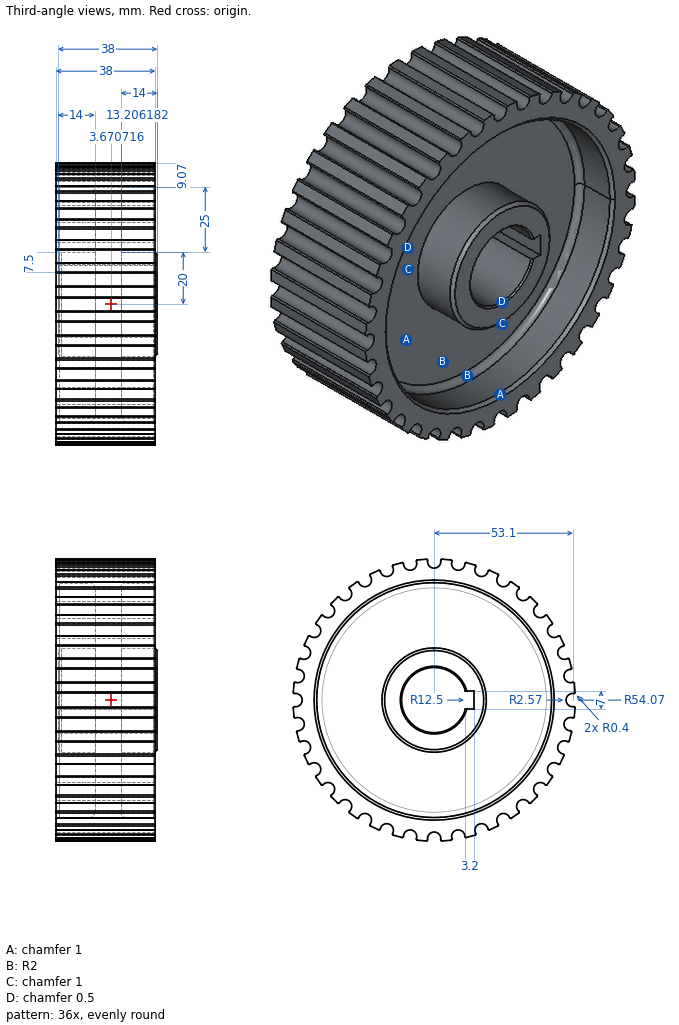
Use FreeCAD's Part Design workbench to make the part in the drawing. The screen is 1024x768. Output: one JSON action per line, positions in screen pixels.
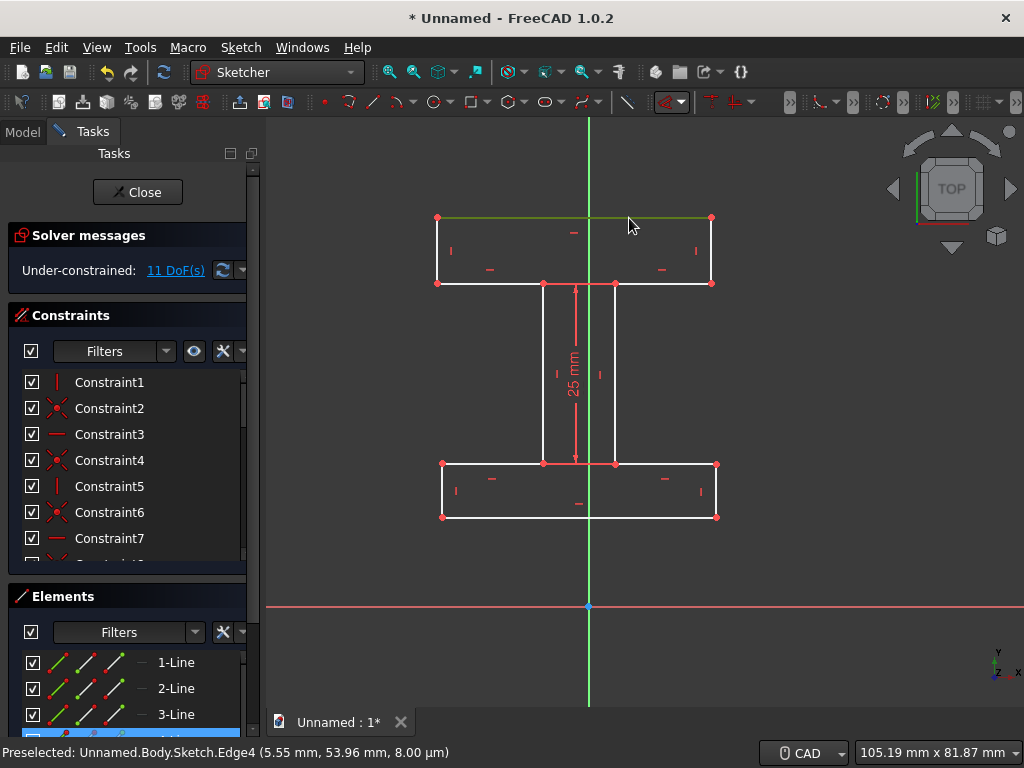
{"action": "left_click", "coordinate": [684, 102]}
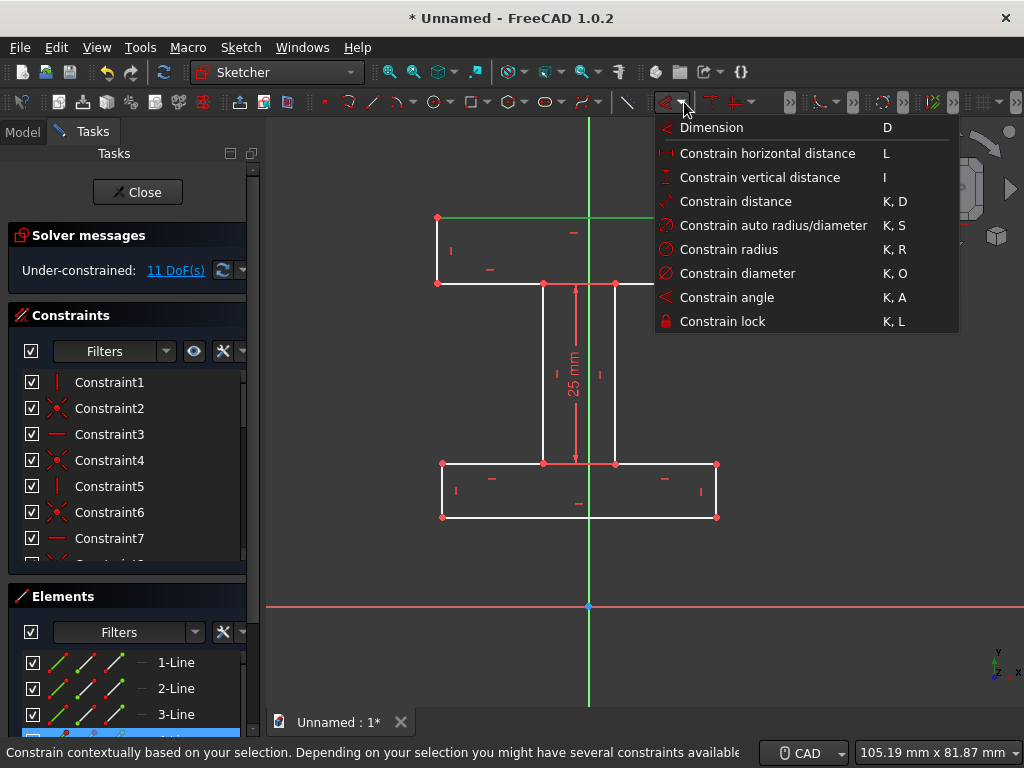
{"action": "left_click", "coordinate": [807, 153]}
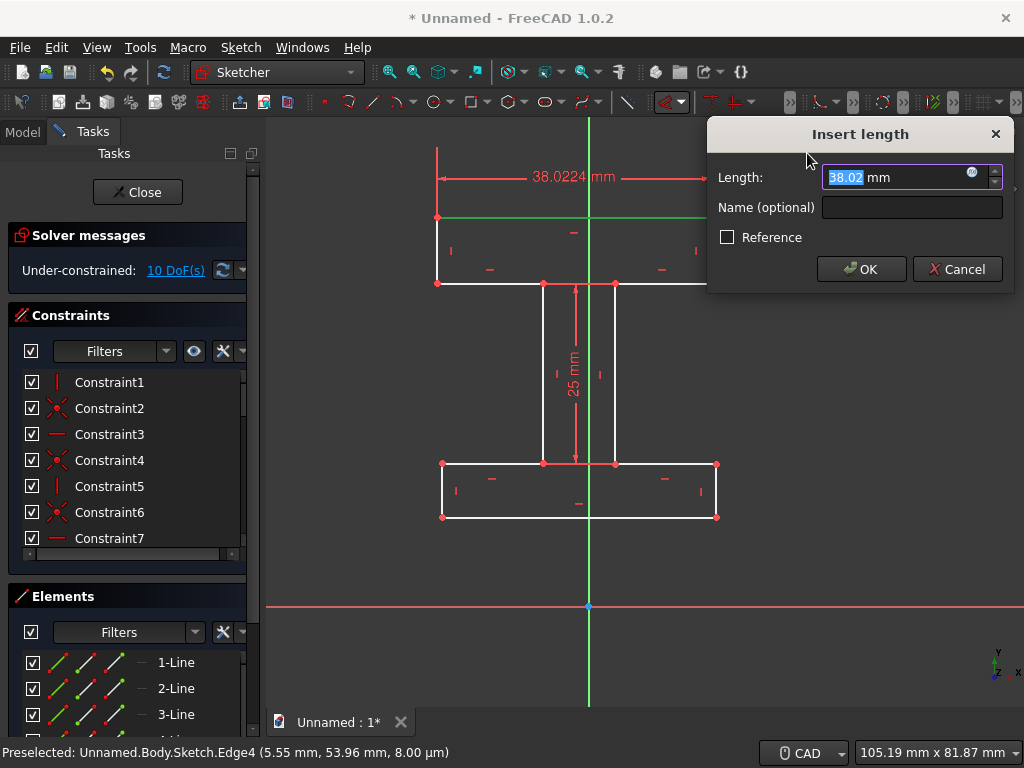
{"action": "type", "text": "38"}
{"action": "key", "text": "Return"}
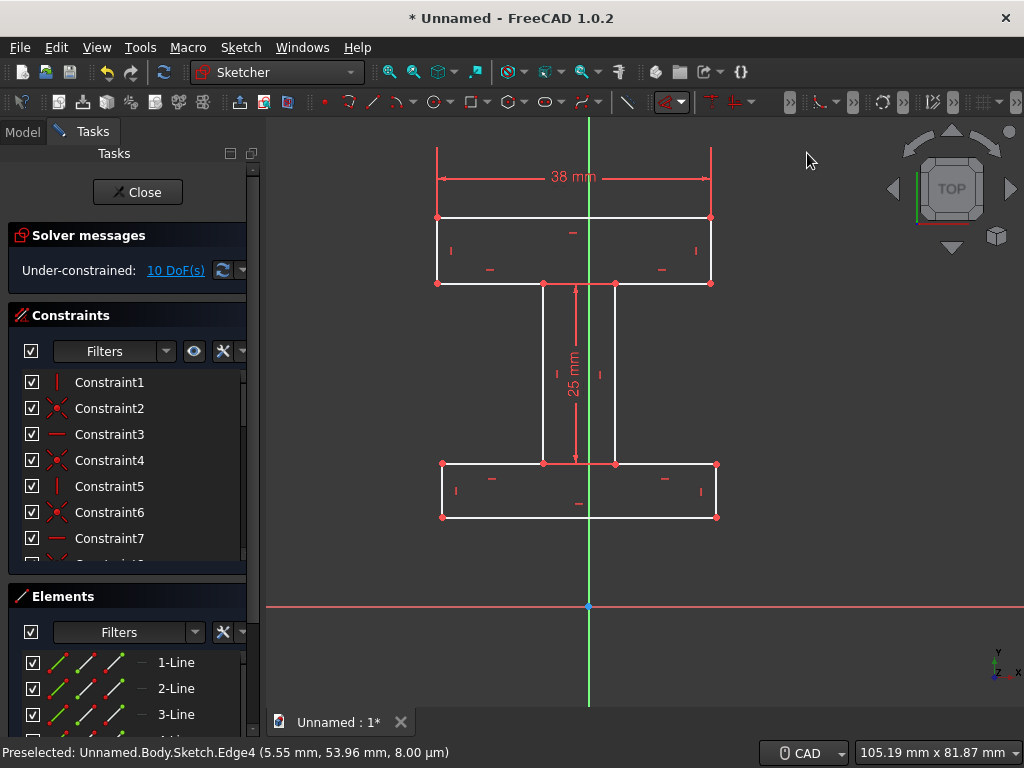
{"action": "left_click", "coordinate": [543, 338]}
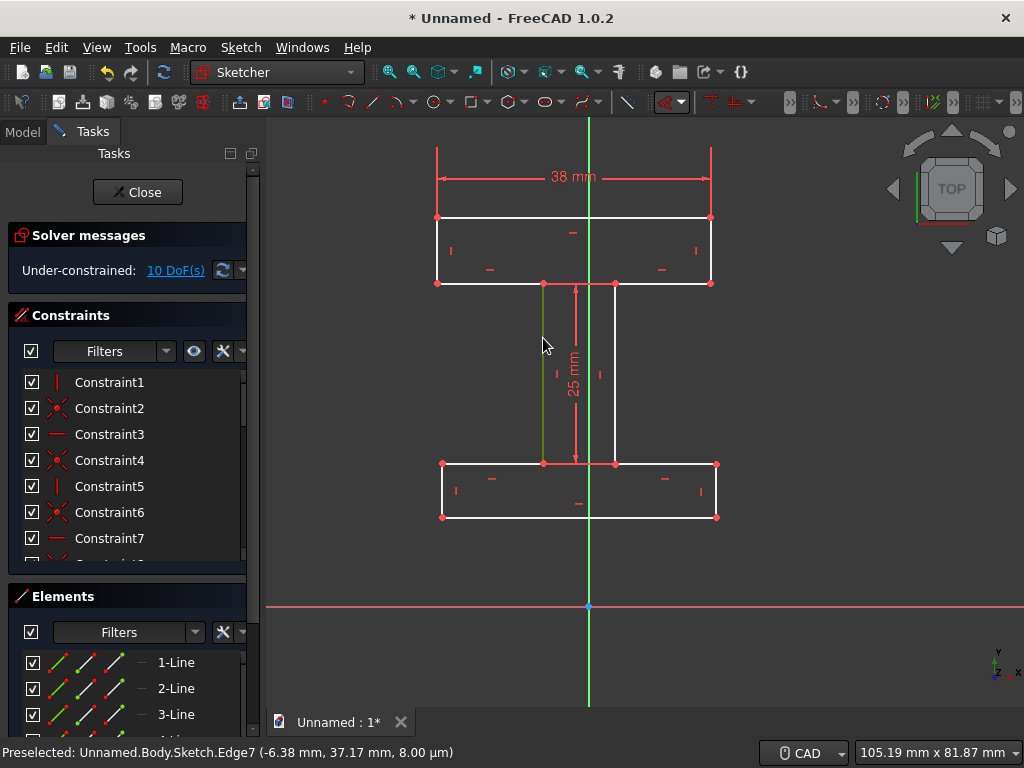
{"action": "left_click", "coordinate": [684, 102]}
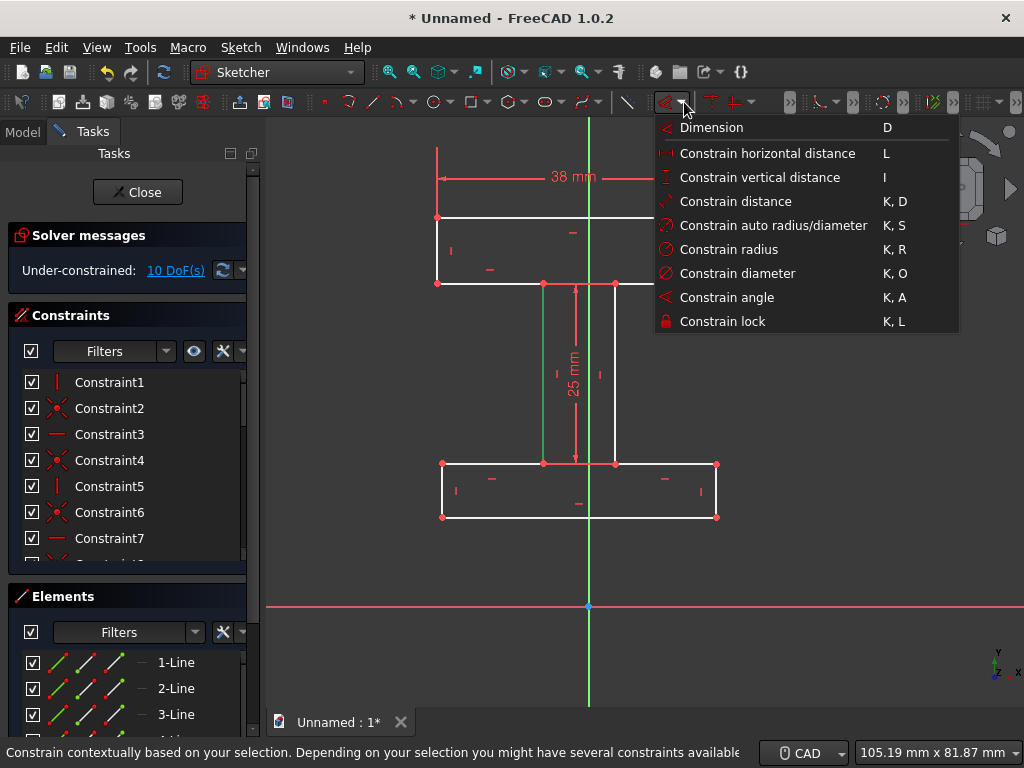
{"action": "left_click", "coordinate": [807, 177]}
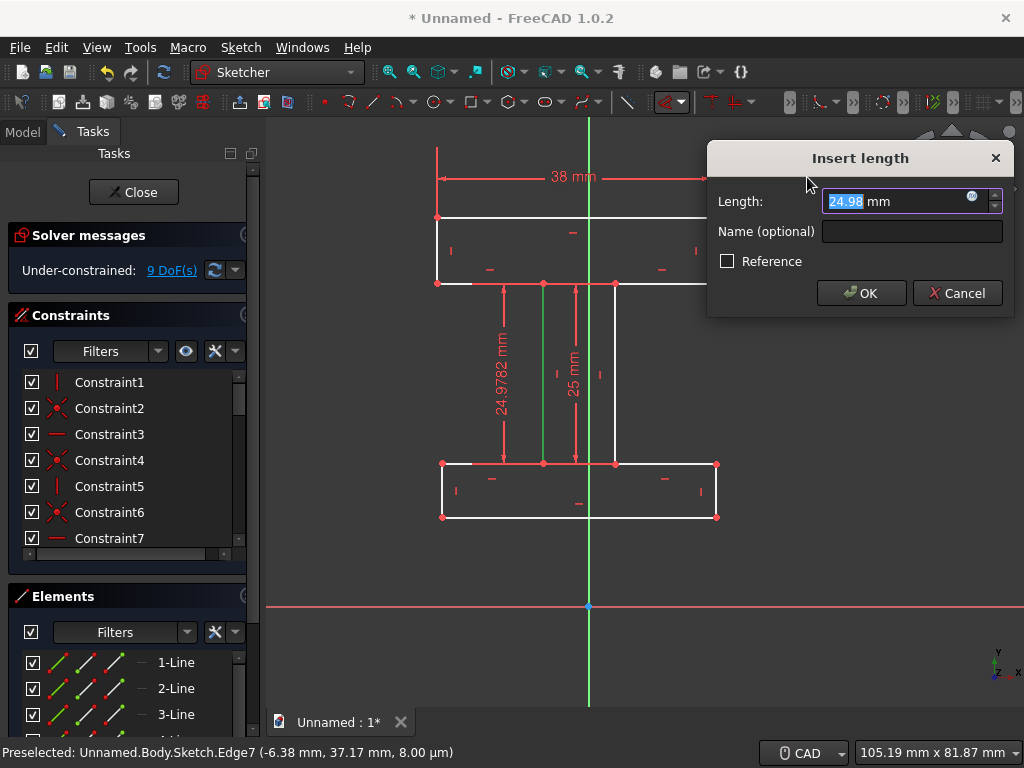
{"action": "type", "text": "25"}
{"action": "key", "text": "Return"}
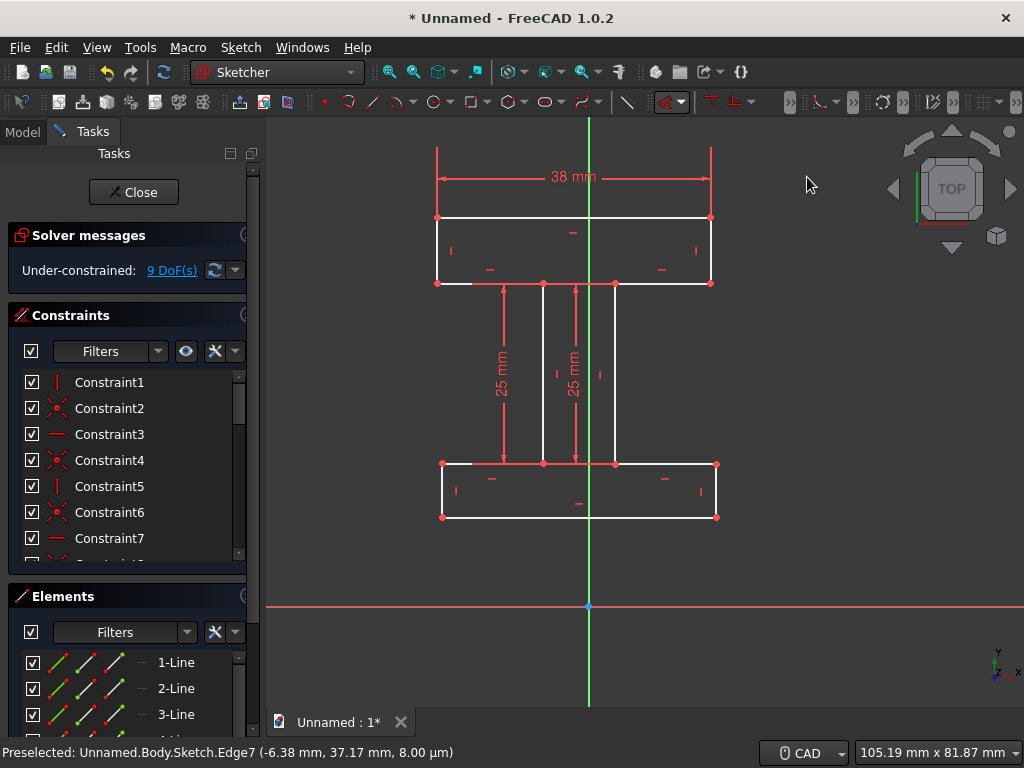
{"action": "left_click", "coordinate": [513, 464]}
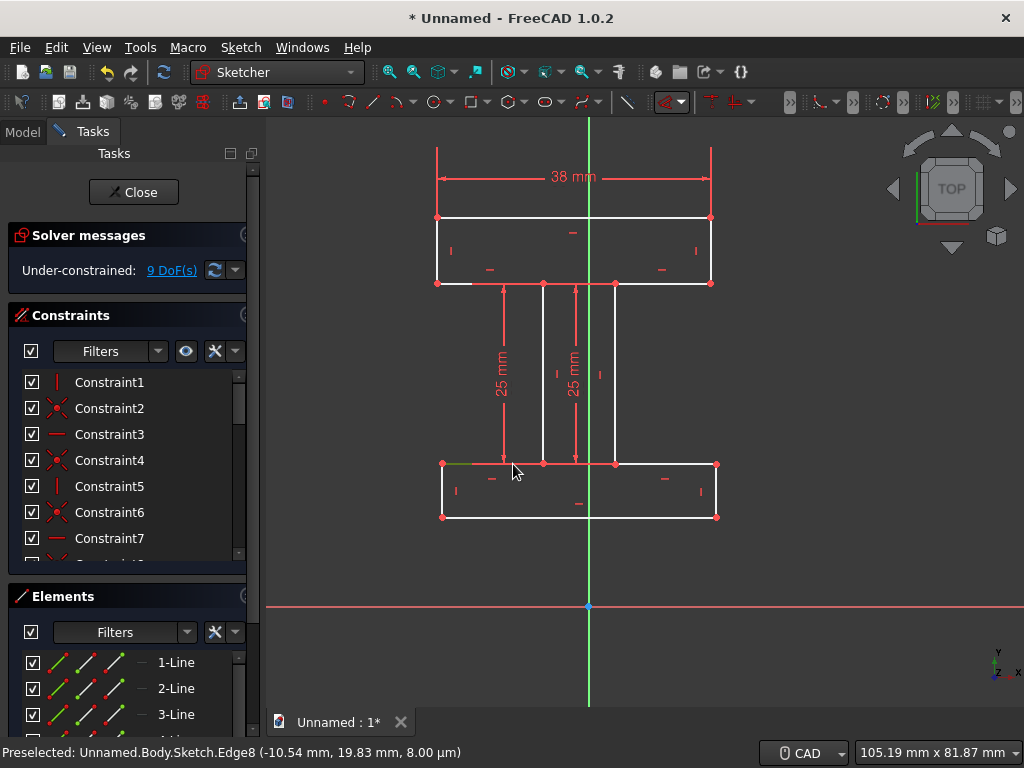
{"action": "left_click", "coordinate": [684, 102]}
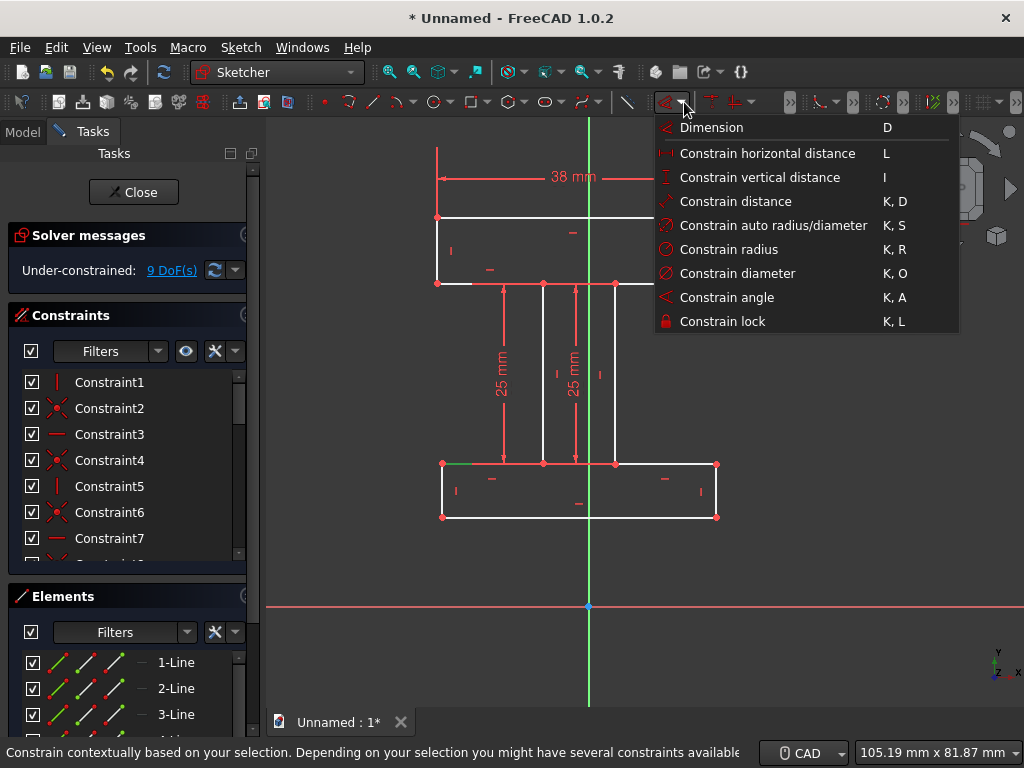
{"action": "left_click", "coordinate": [807, 153]}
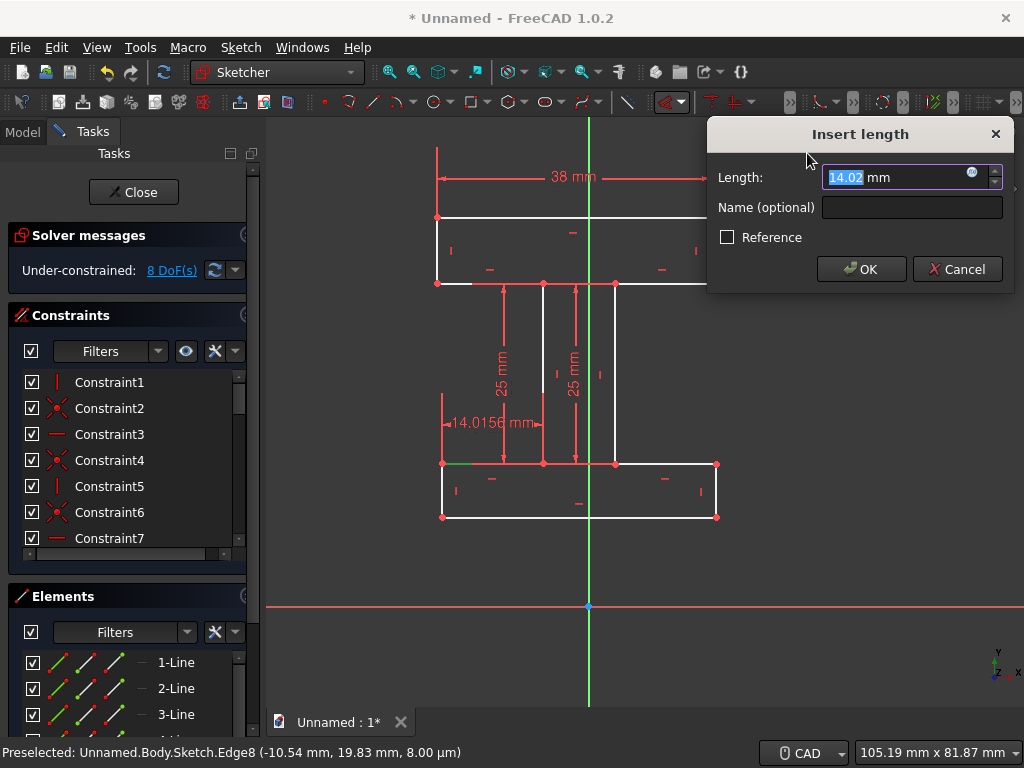
{"action": "type", "text": "14"}
{"action": "key", "text": "Return"}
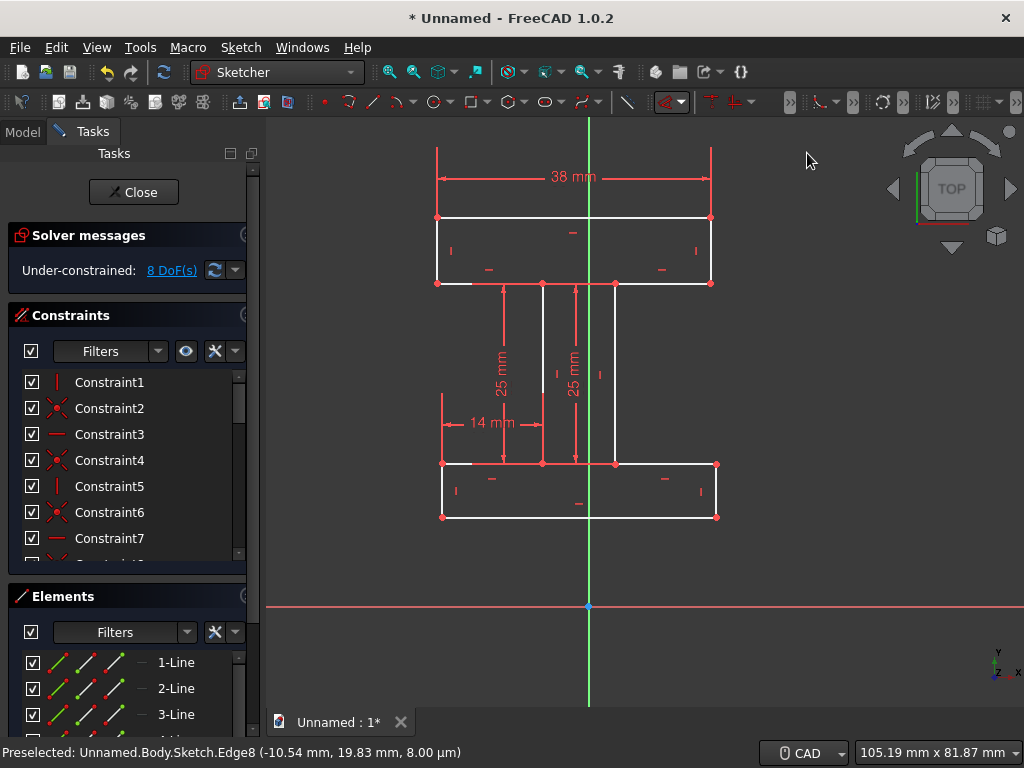
{"action": "left_click", "coordinate": [524, 518]}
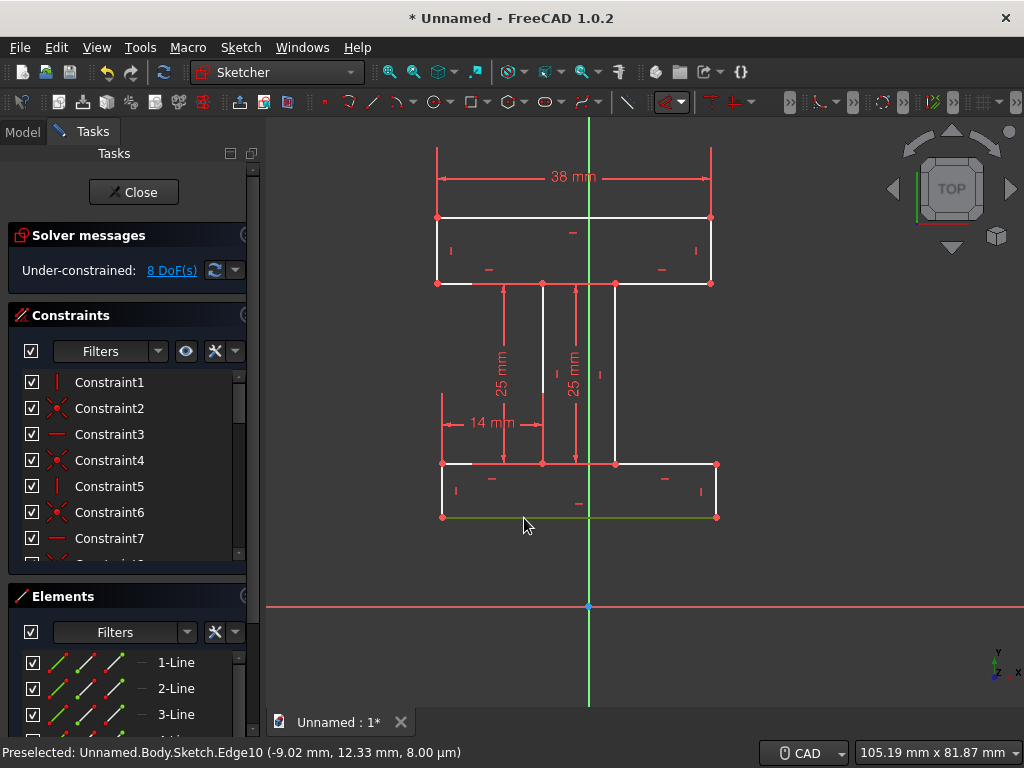
{"action": "left_click", "coordinate": [684, 102]}